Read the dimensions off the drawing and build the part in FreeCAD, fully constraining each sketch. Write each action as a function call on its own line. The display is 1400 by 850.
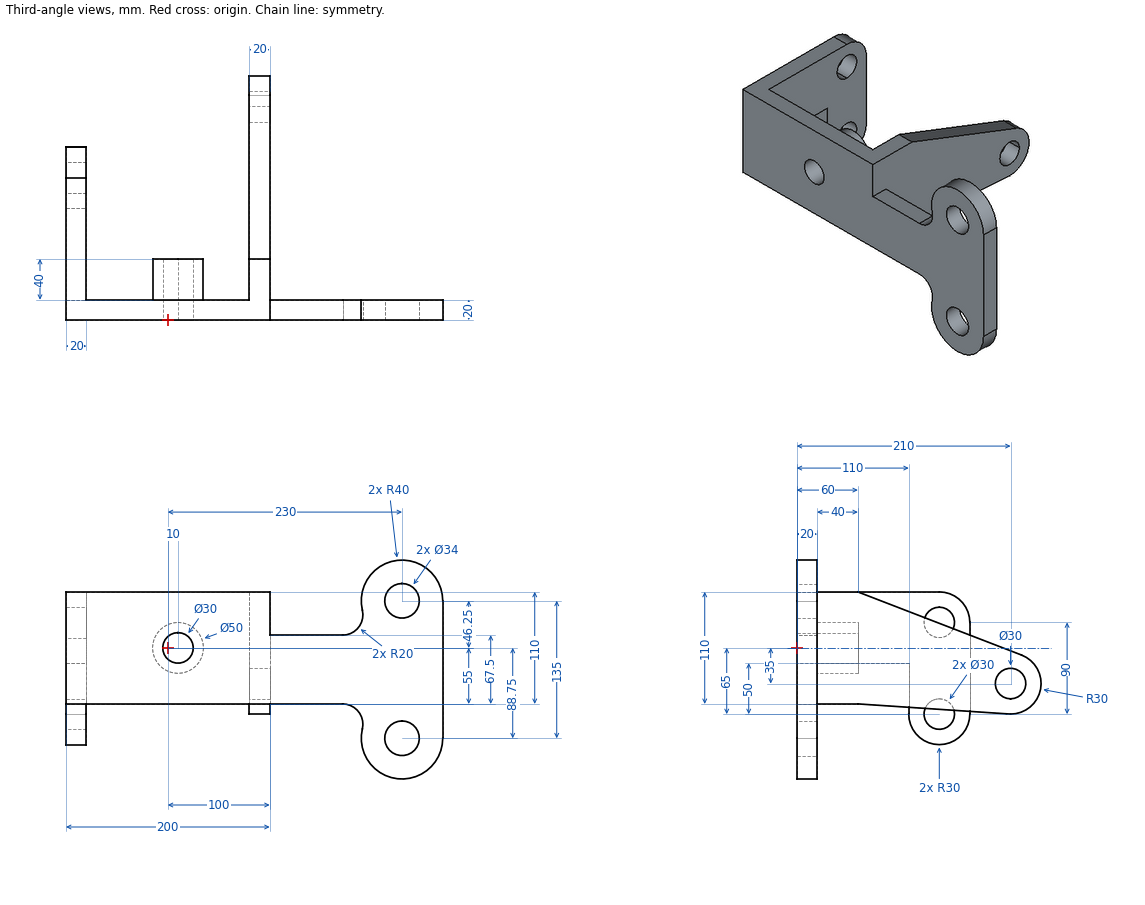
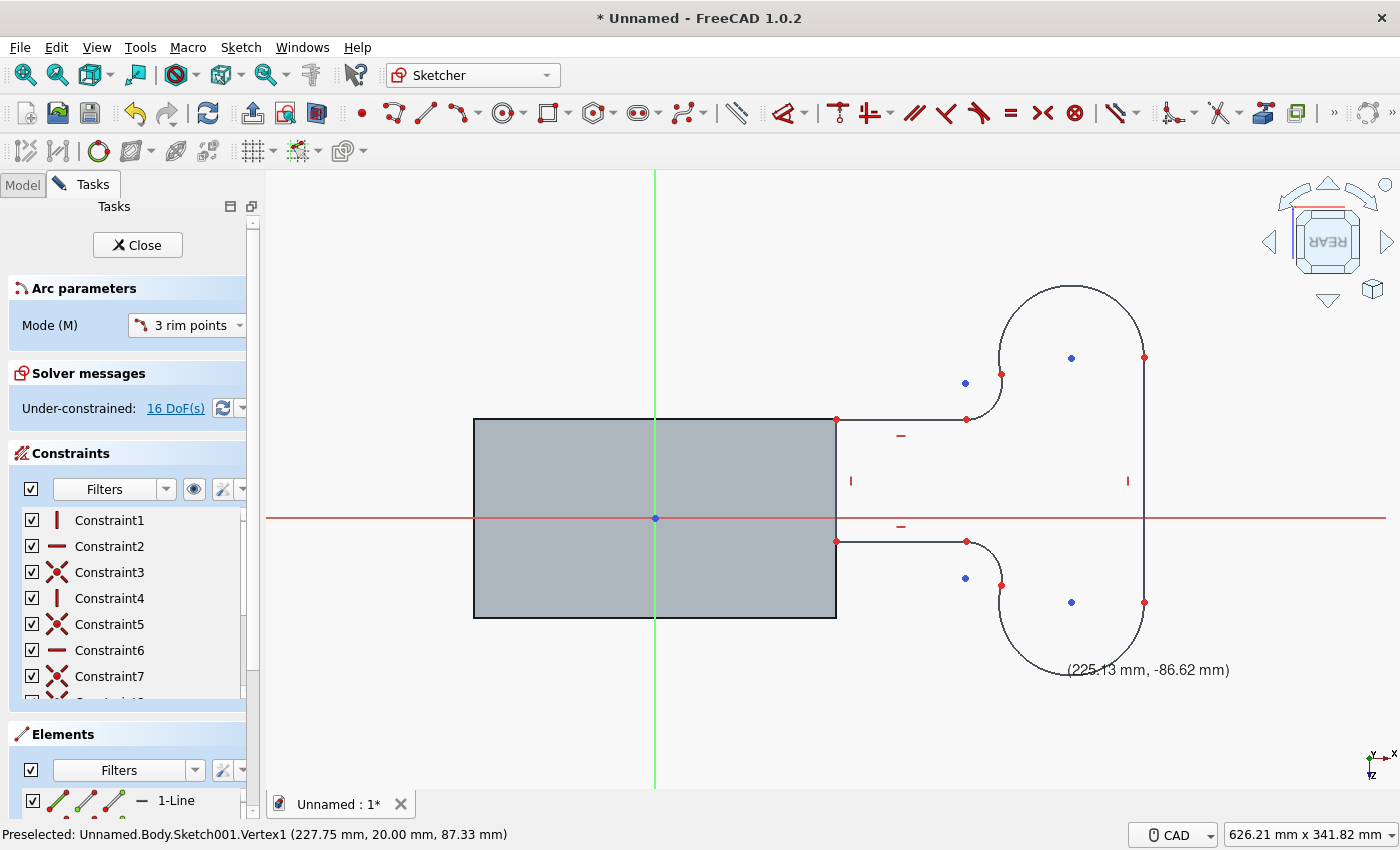
key(g)
key(c)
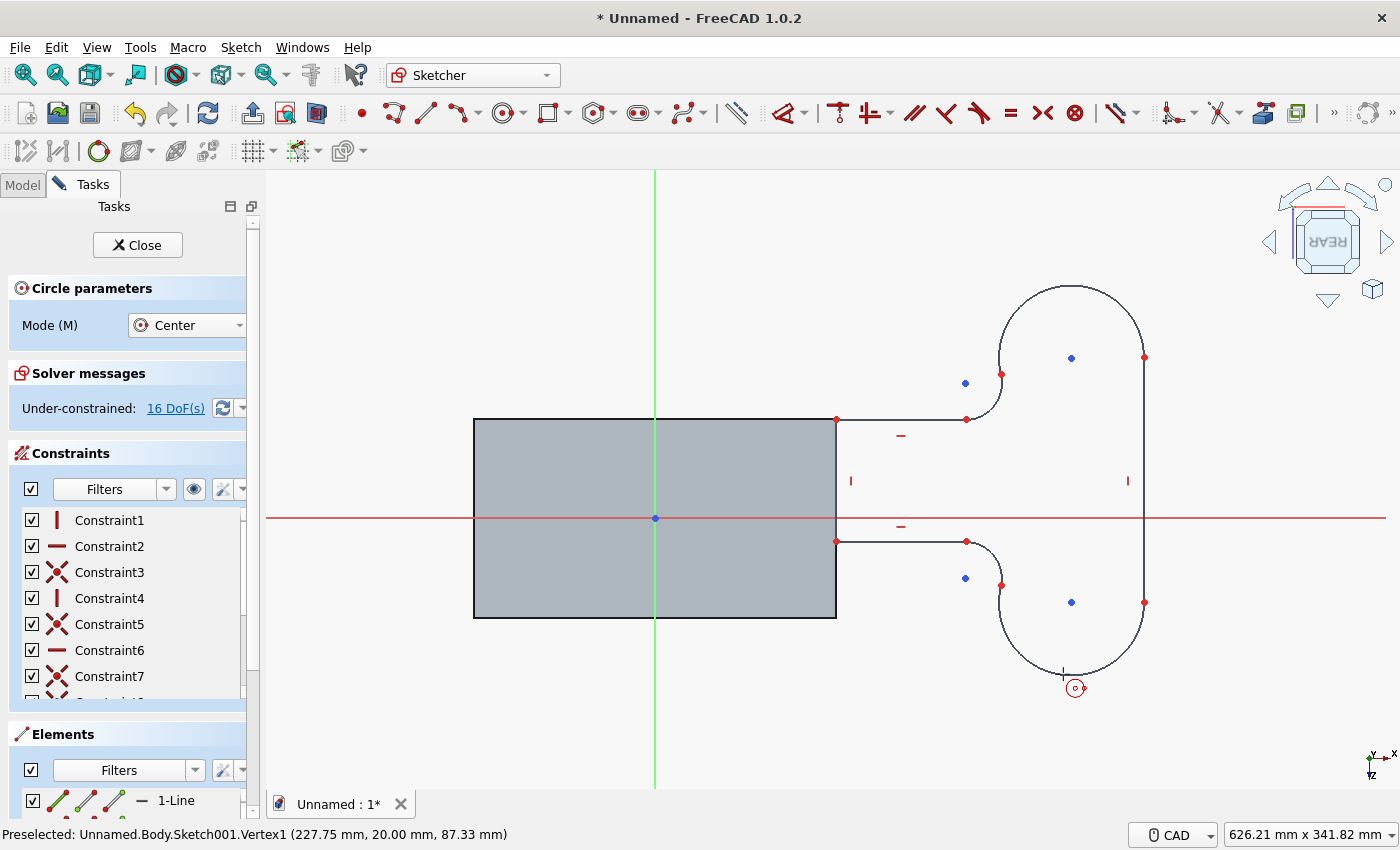
click(1072, 602)
click(1094, 580)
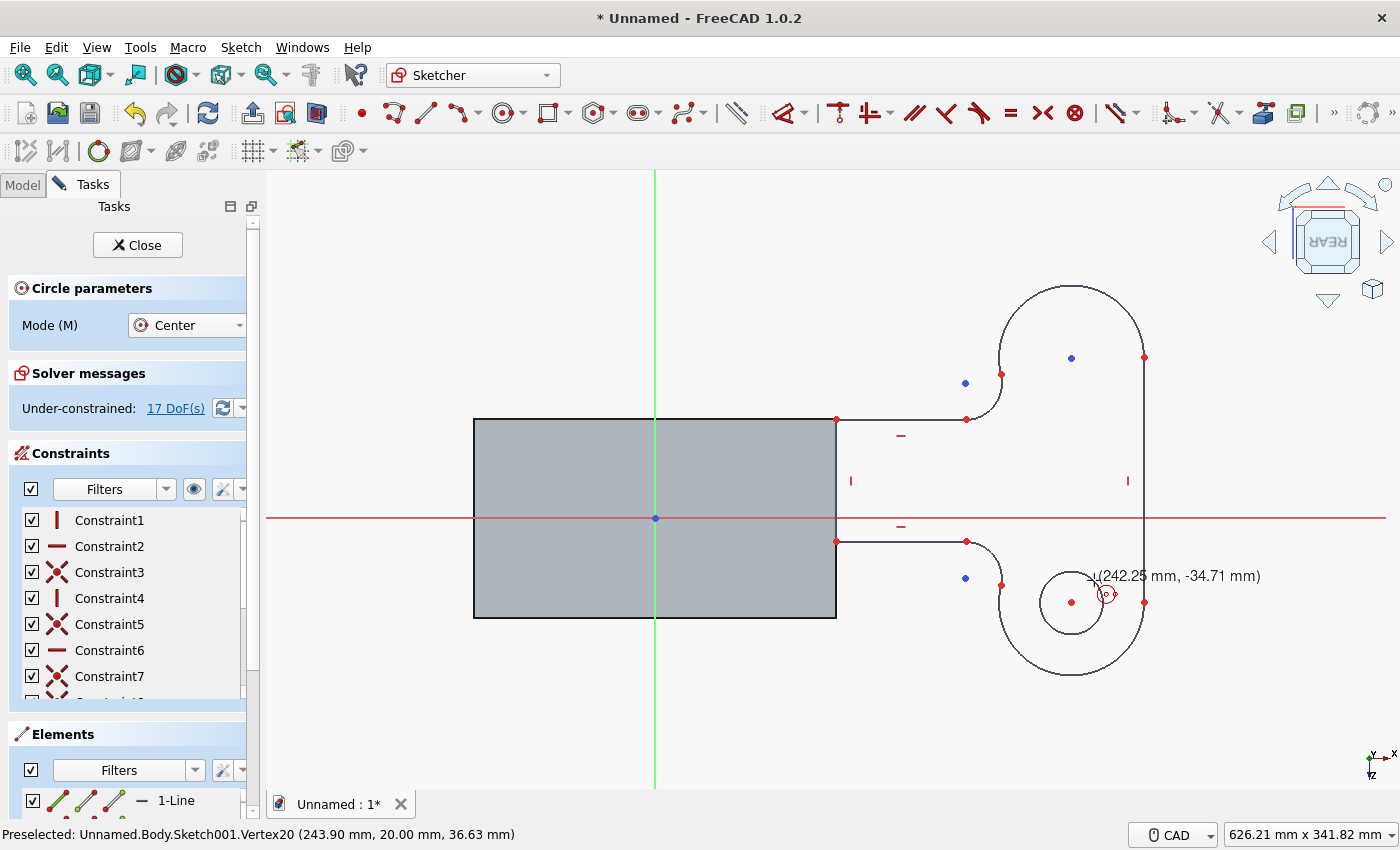
click(1072, 357)
click(1094, 336)
key(Escape)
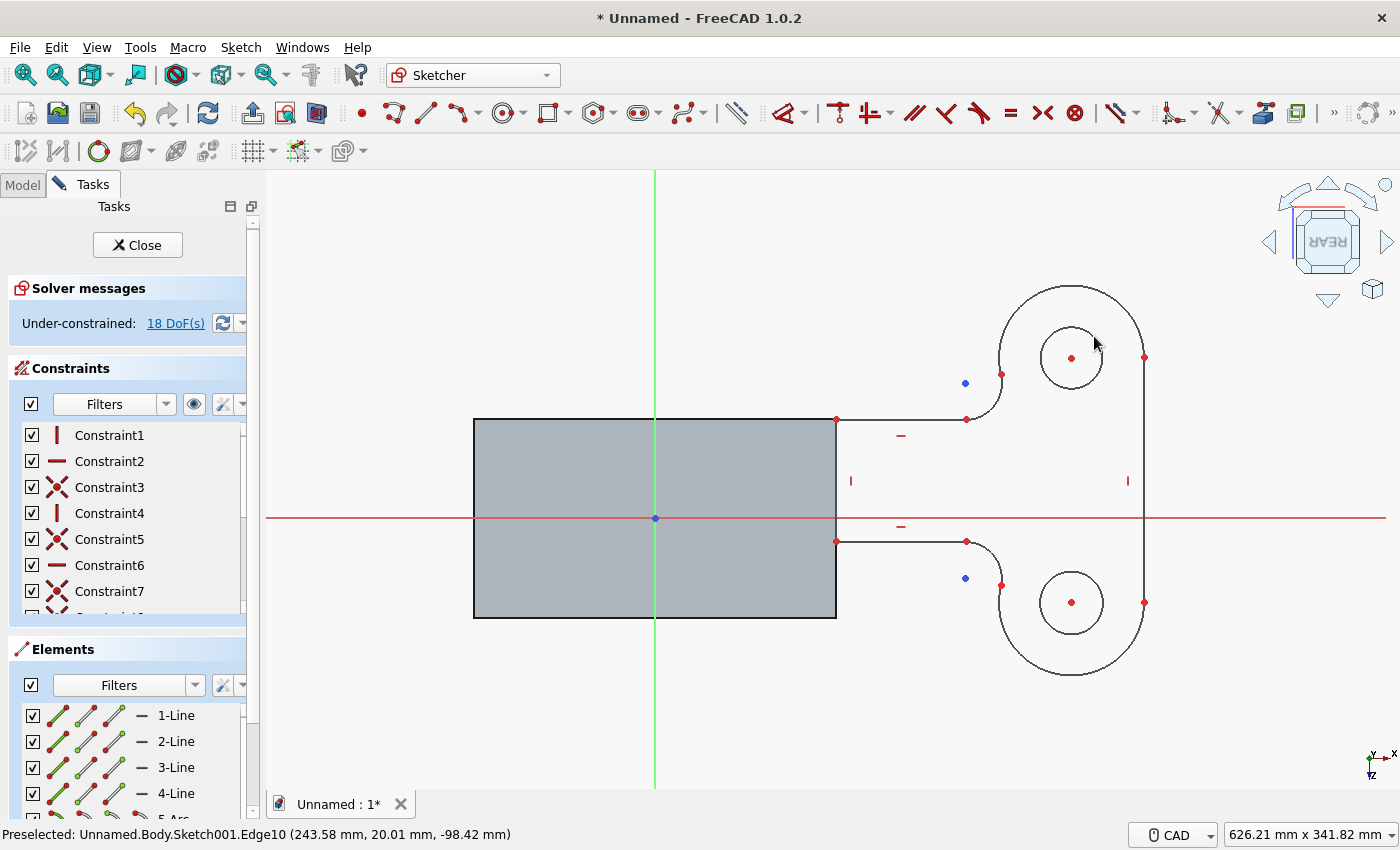
click(927, 420)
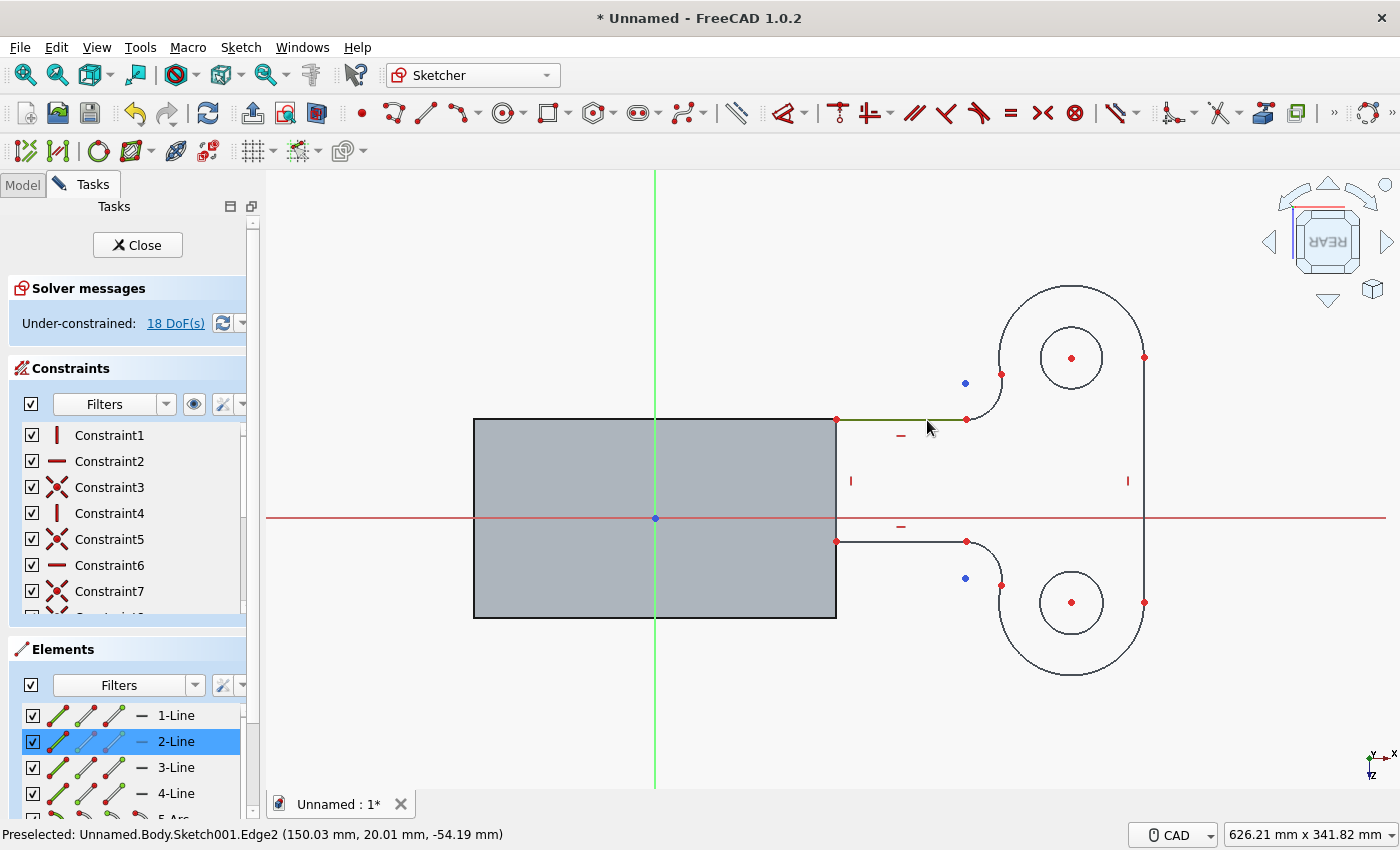
click(985, 414)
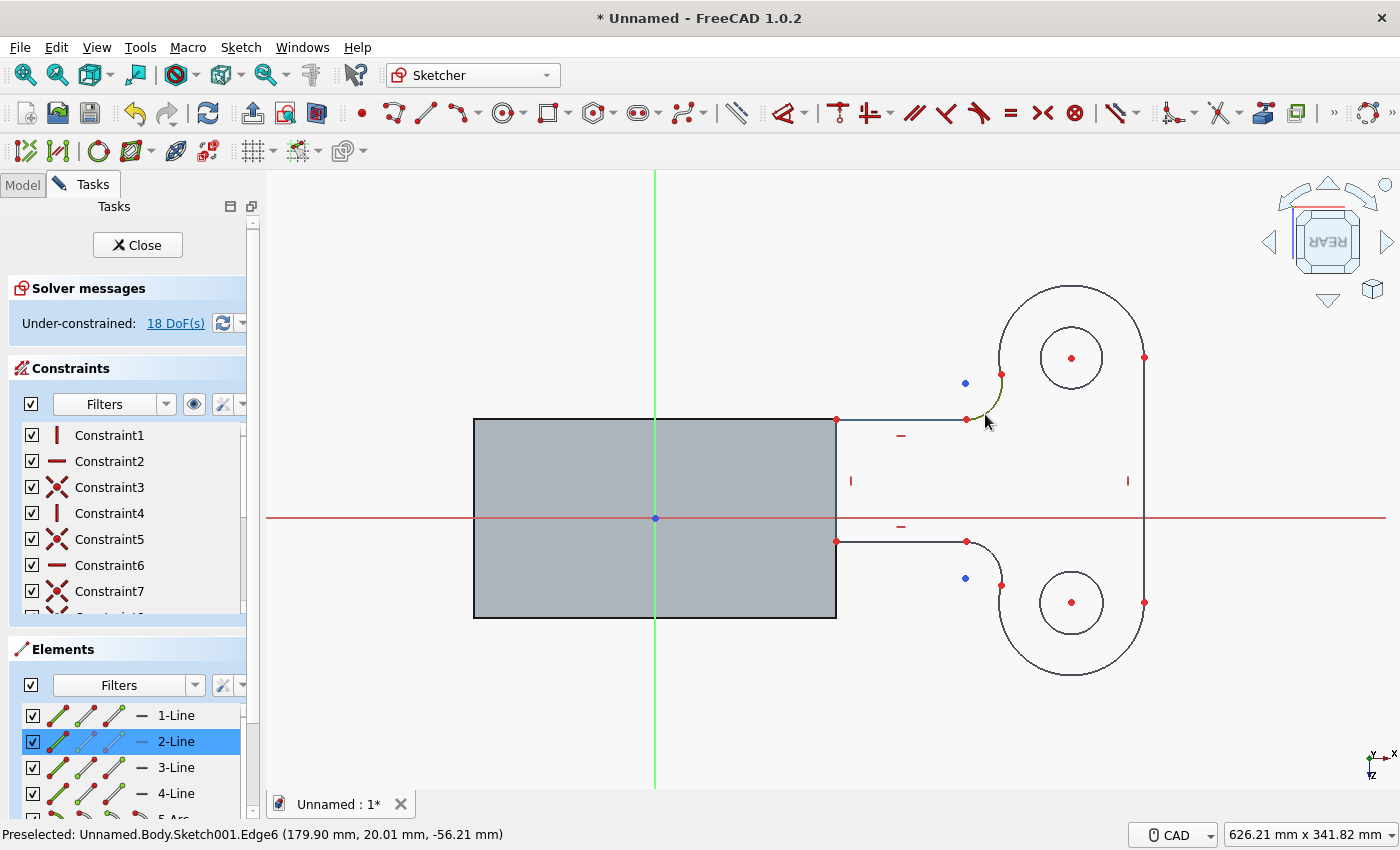
click(980, 114)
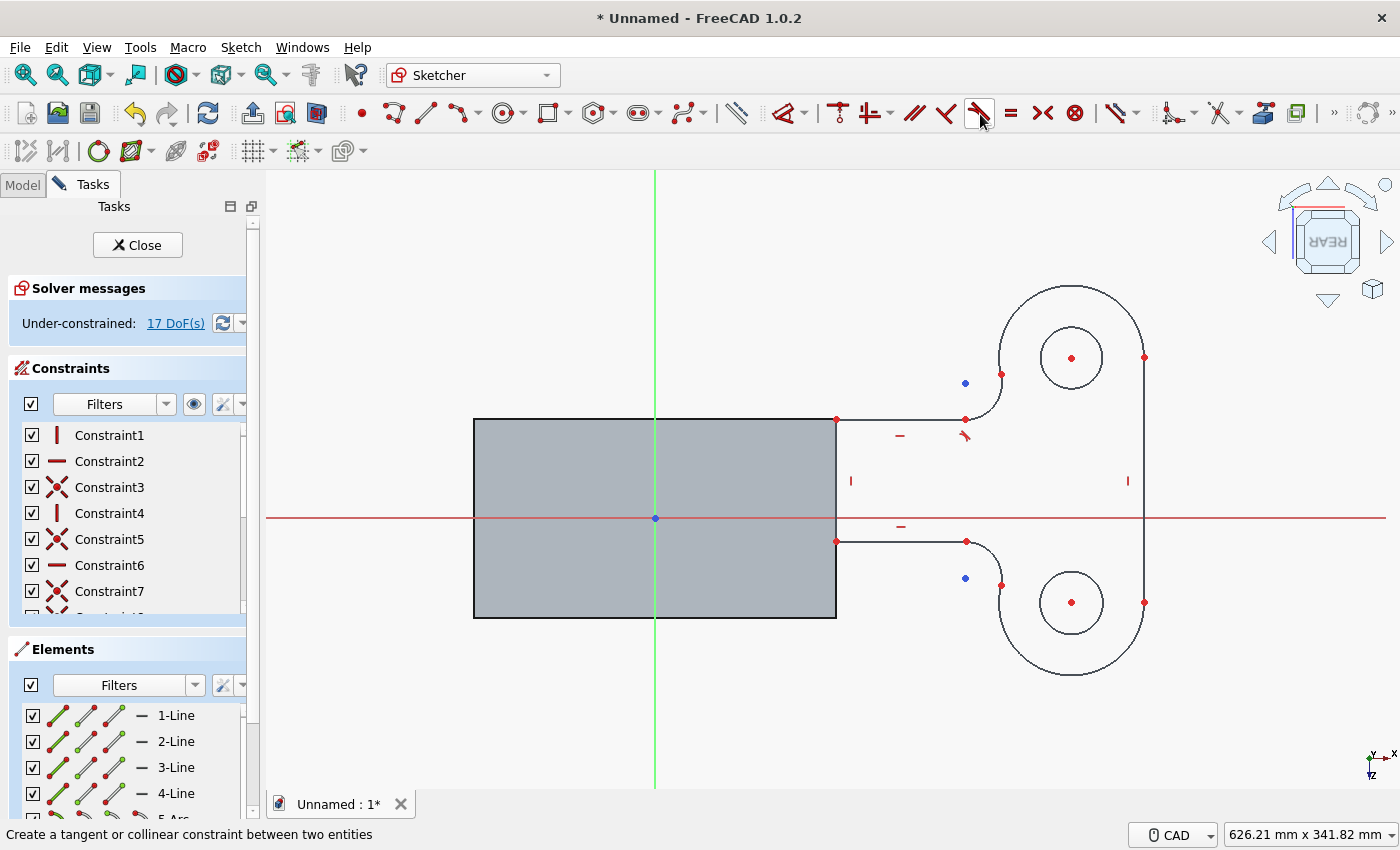
click(875, 542)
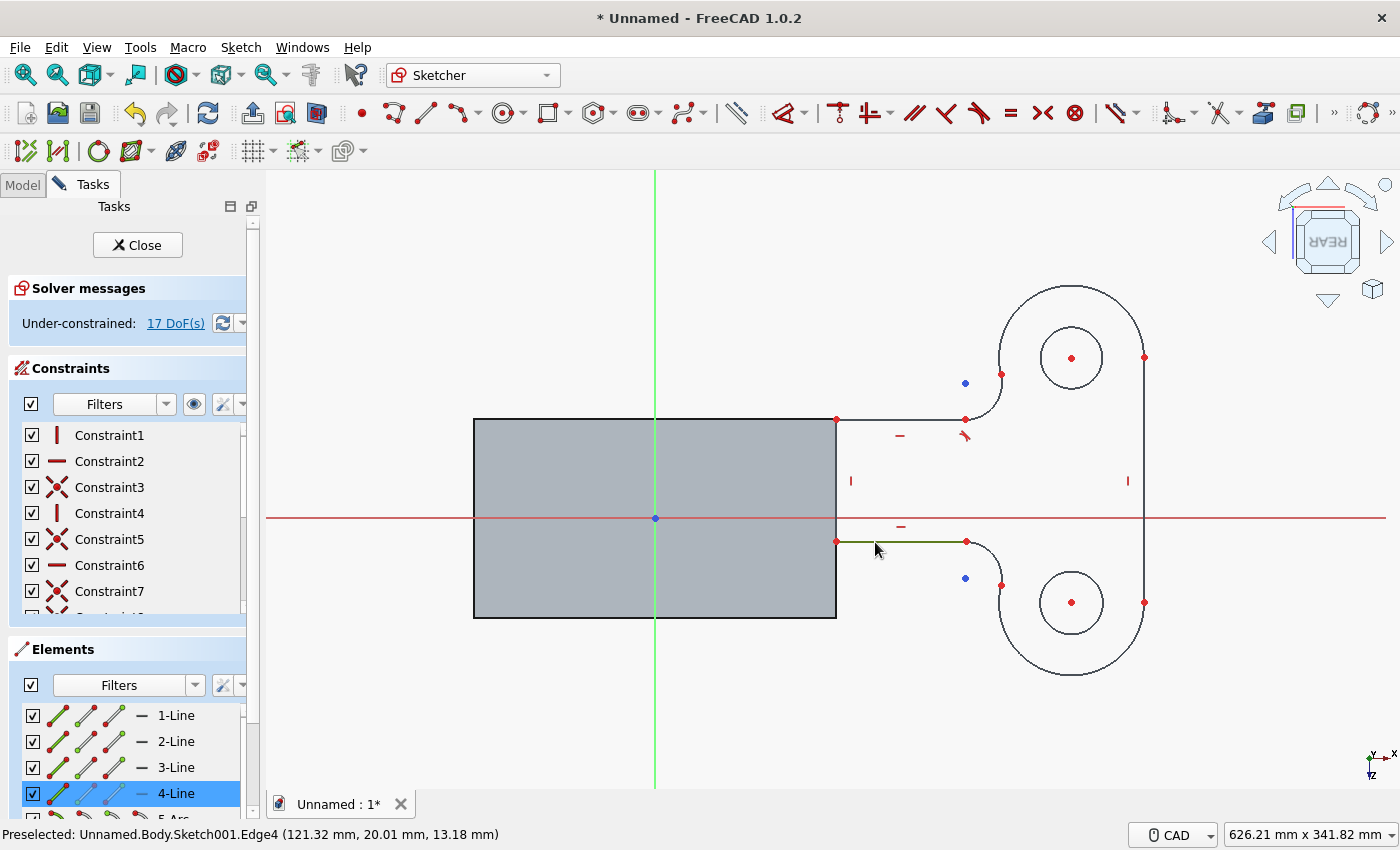
click(1000, 567)